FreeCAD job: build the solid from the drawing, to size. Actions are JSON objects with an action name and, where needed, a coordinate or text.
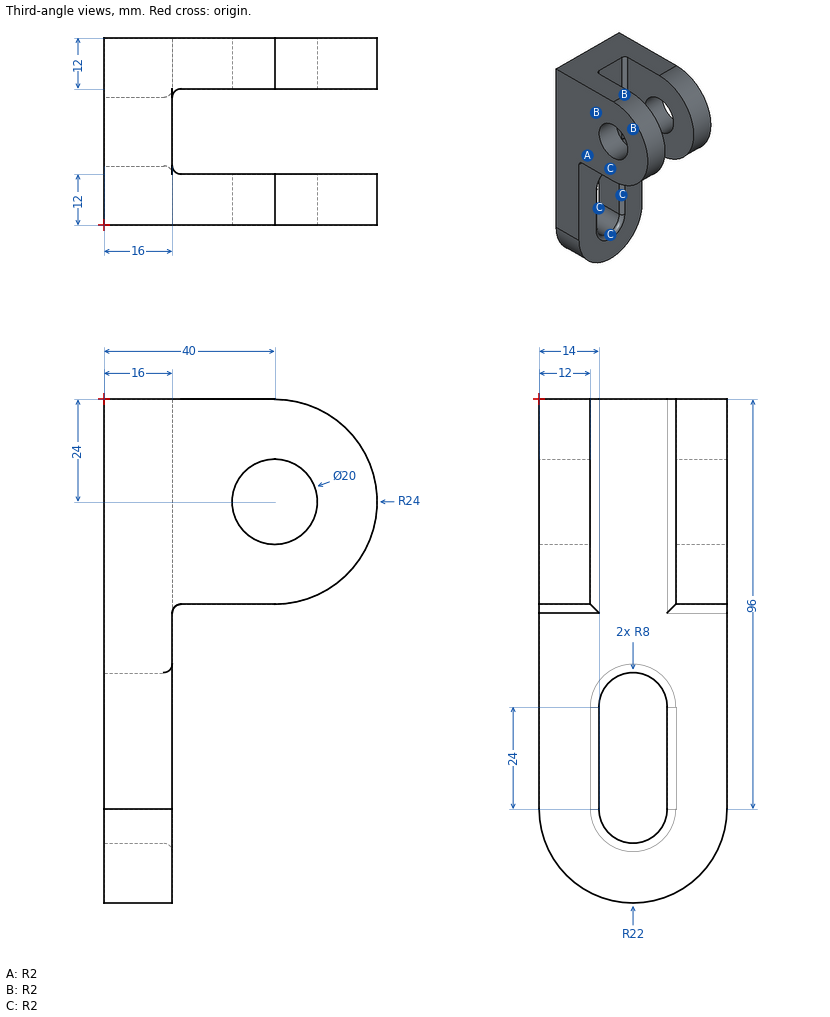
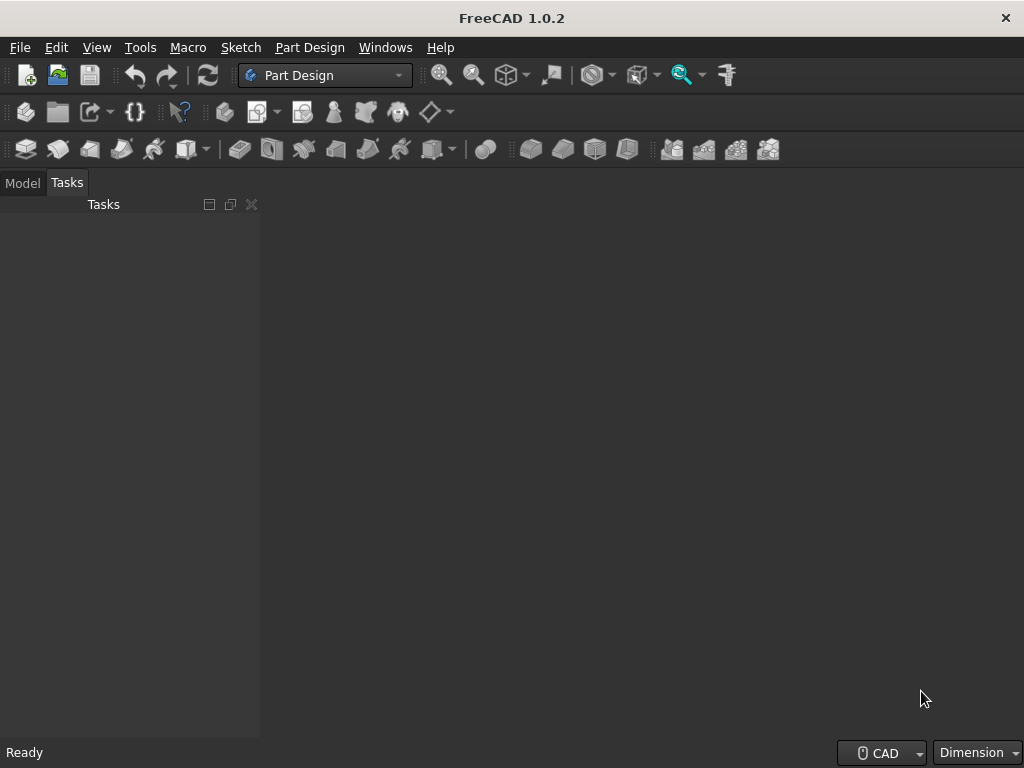
{"action": "left_click", "coordinate": [26, 76]}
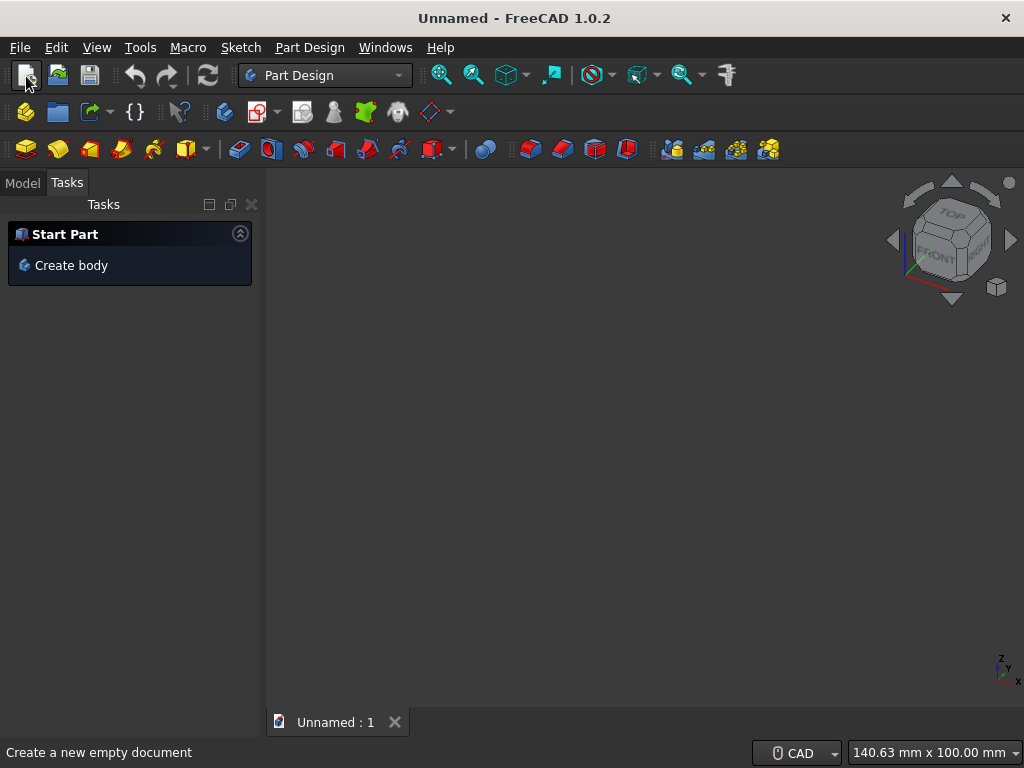
{"action": "left_click", "coordinate": [258, 112]}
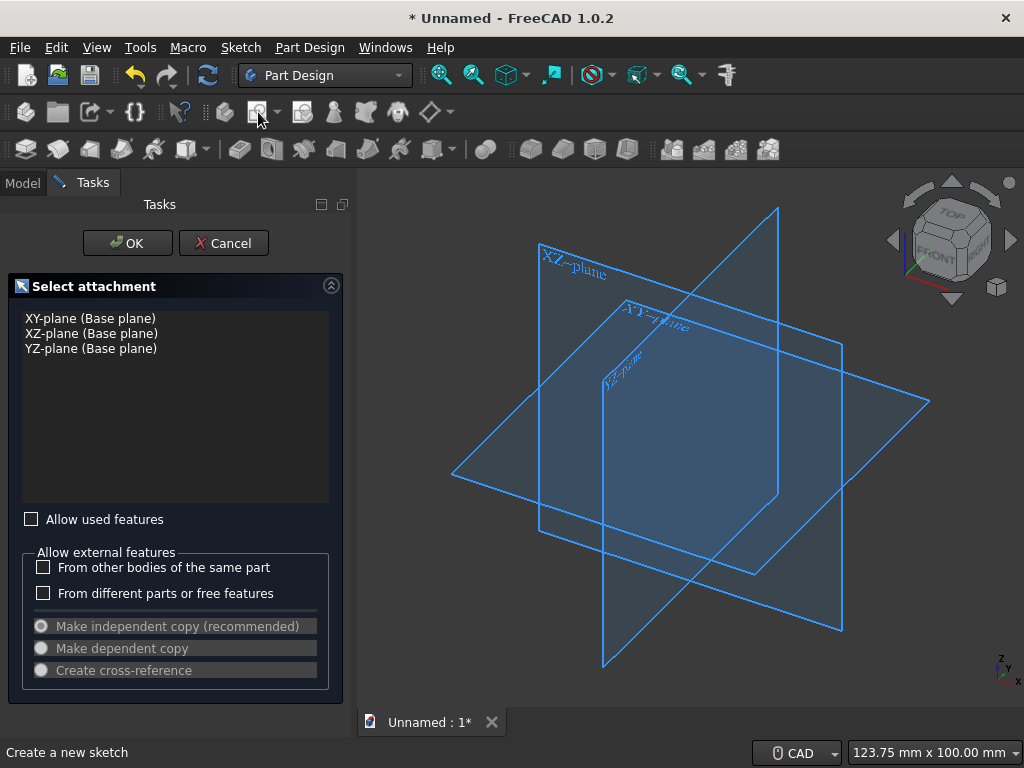
{"action": "left_click", "coordinate": [82, 348]}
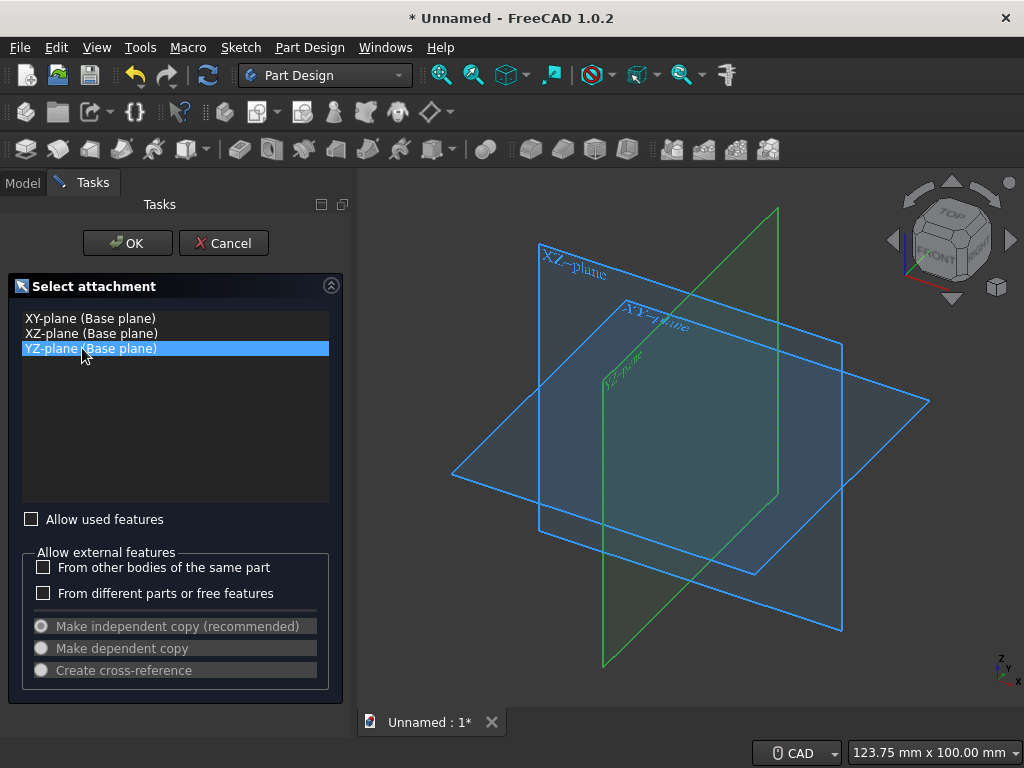
{"action": "left_click", "coordinate": [128, 243]}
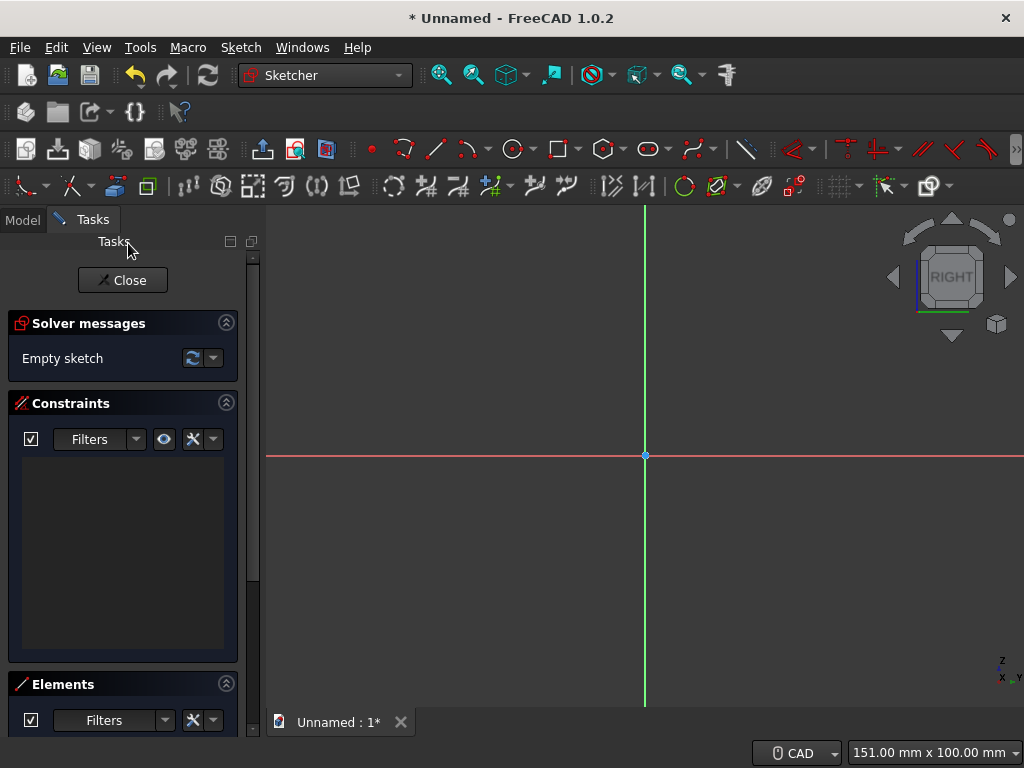
{"action": "scroll", "coordinate": [430, 233], "scroll_direction": "down", "scroll_amount": 4}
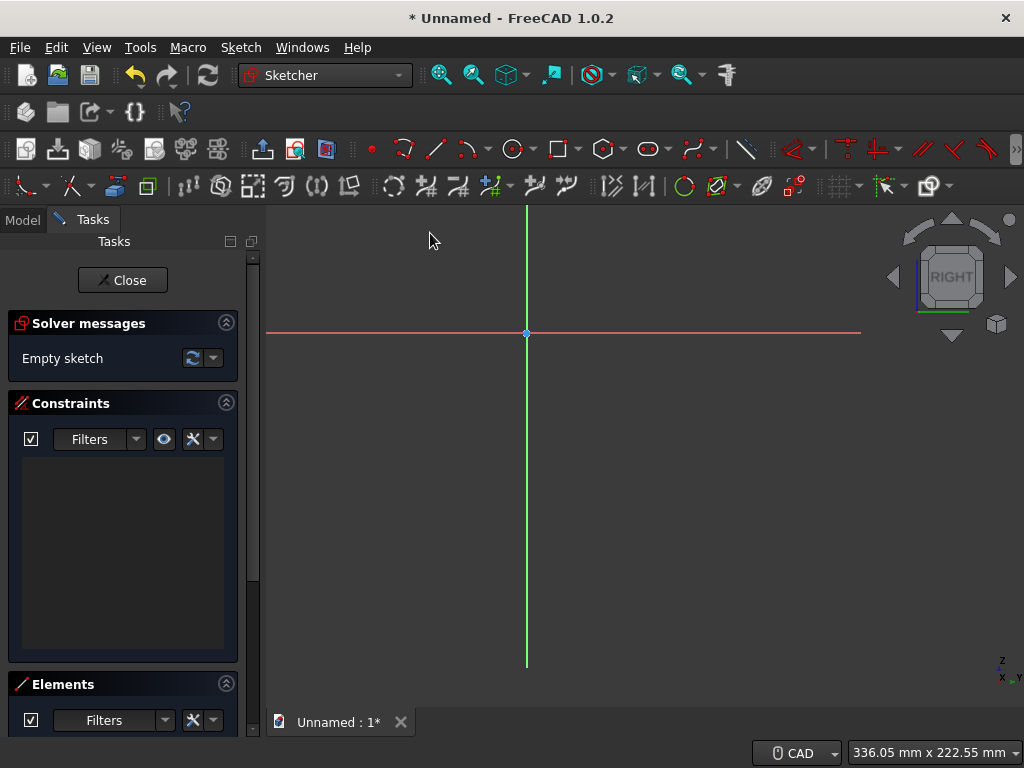
{"action": "left_click", "coordinate": [404, 150]}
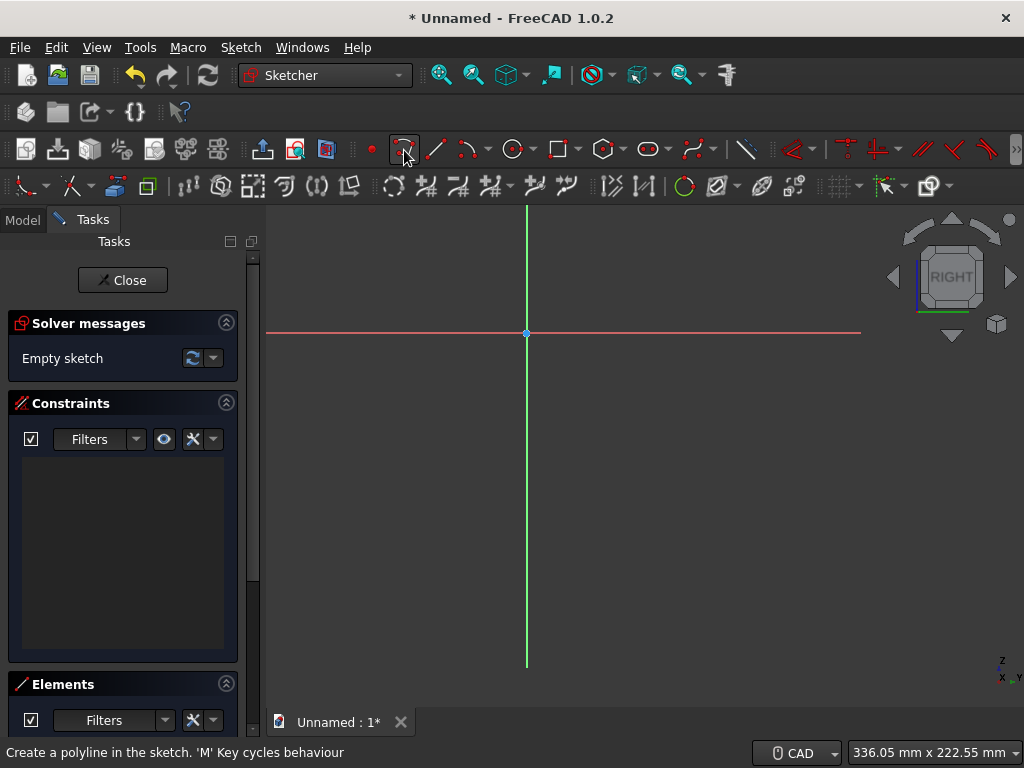
{"action": "left_click", "coordinate": [626, 550]}
{"action": "left_click", "coordinate": [626, 333]}
{"action": "left_click", "coordinate": [527, 333]}
{"action": "left_click", "coordinate": [536, 550]}
{"action": "right_click", "coordinate": [536, 550]}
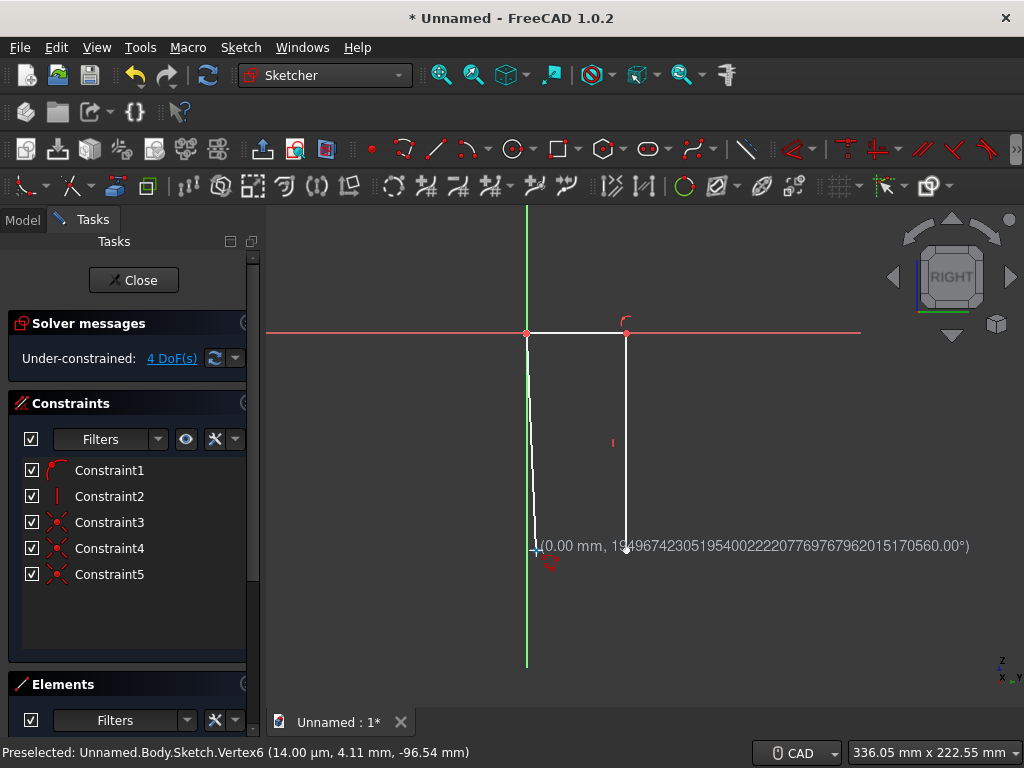
{"action": "left_click", "coordinate": [490, 150]}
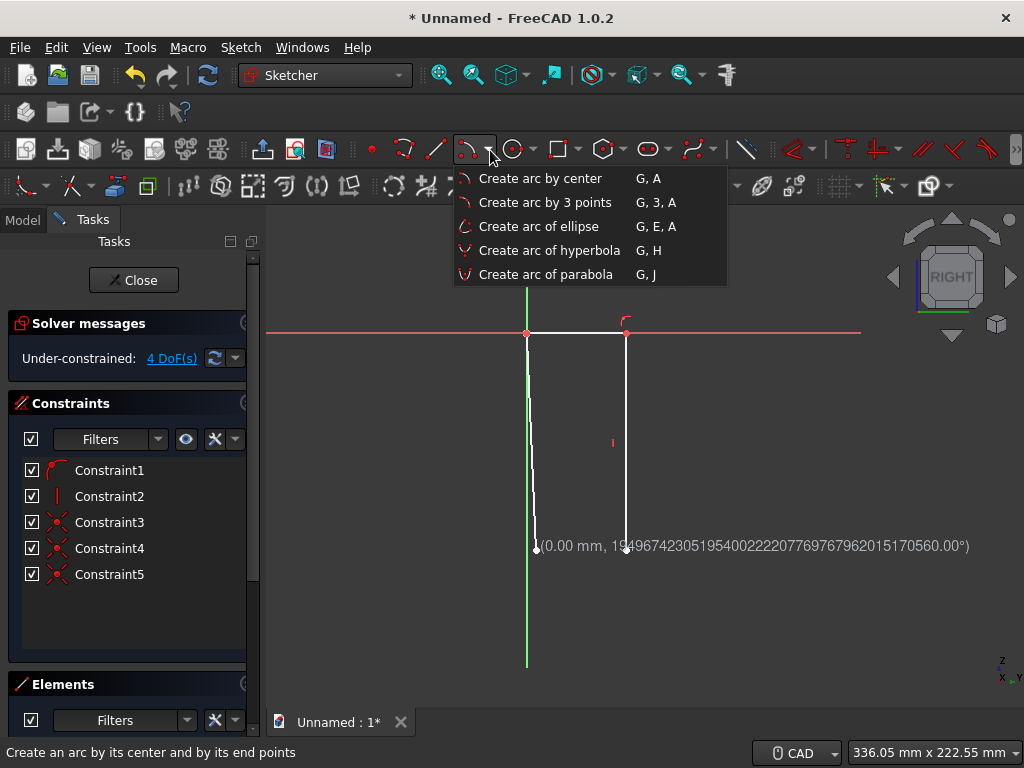
{"action": "left_click", "coordinate": [590, 202]}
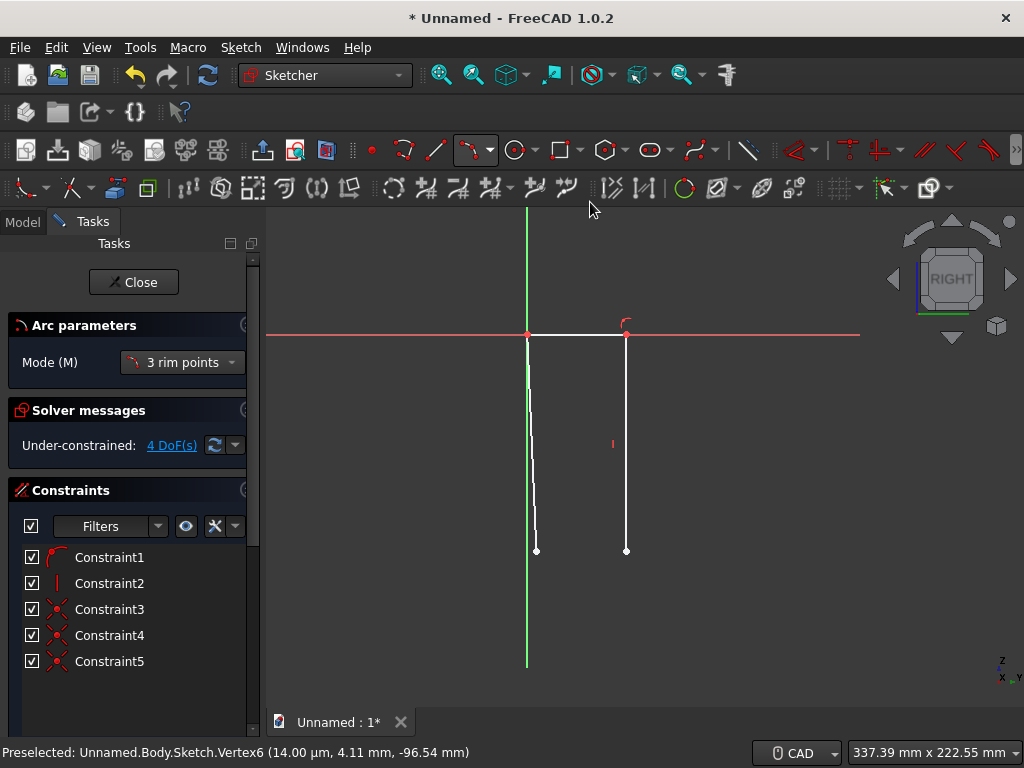
{"action": "left_click", "coordinate": [536, 552]}
{"action": "left_click", "coordinate": [626, 552]}
{"action": "left_click", "coordinate": [577, 600]}
{"action": "key", "text": "Escape"}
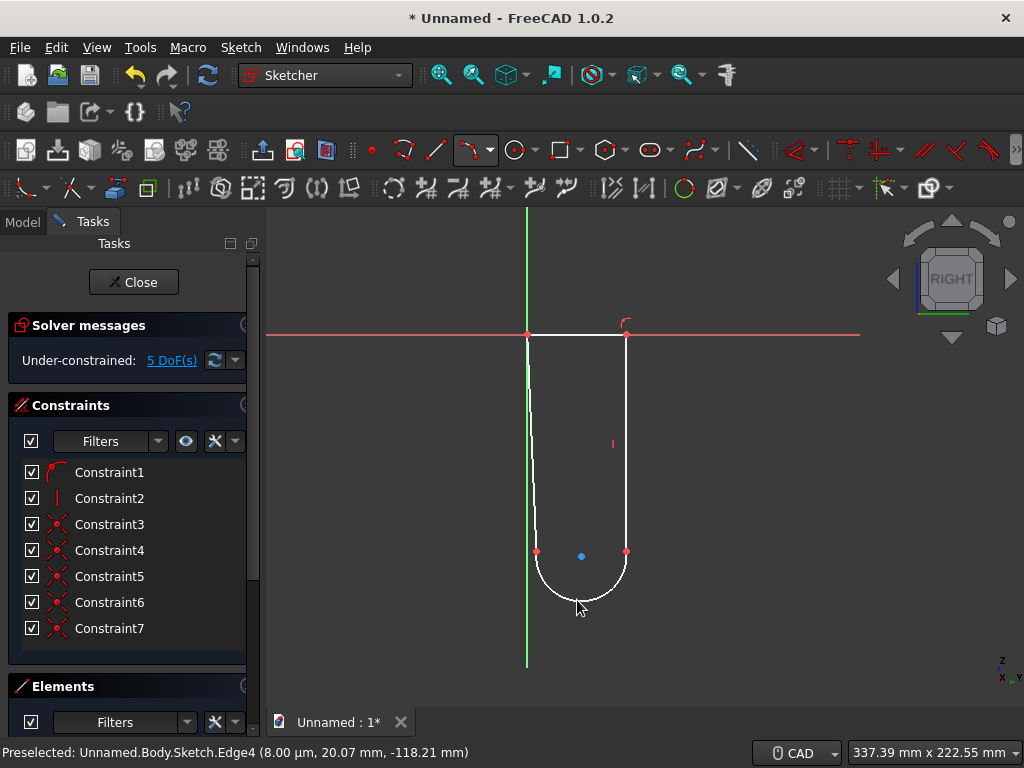
{"action": "left_click", "coordinate": [626, 487]}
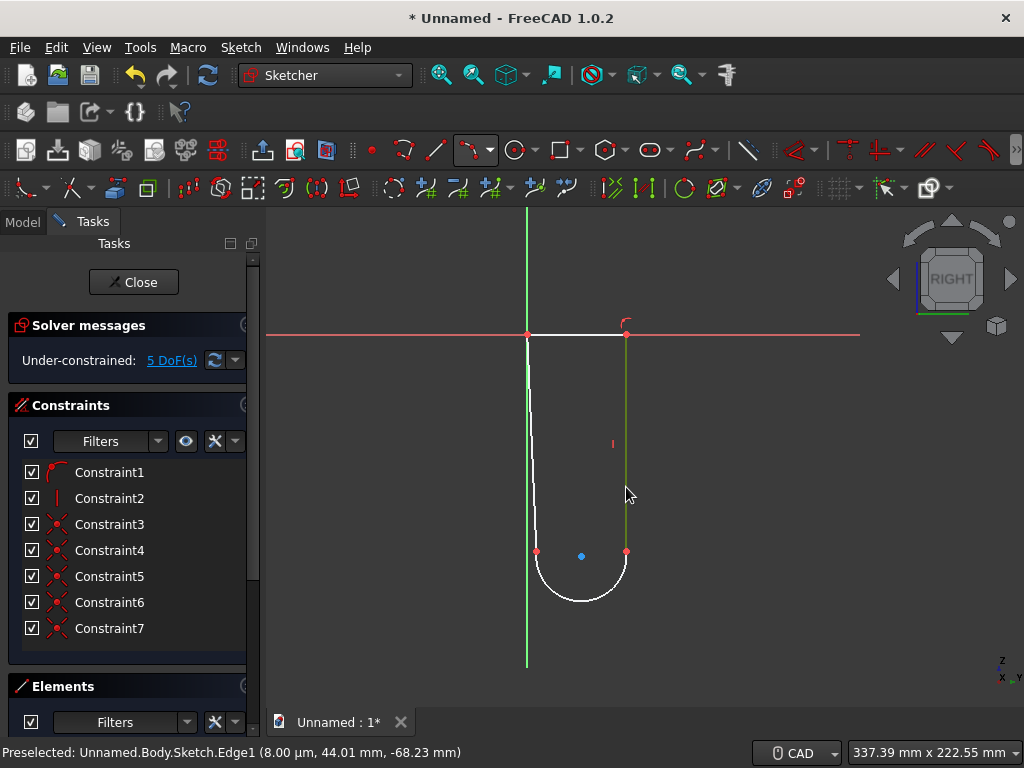
{"action": "left_click", "coordinate": [553, 592]}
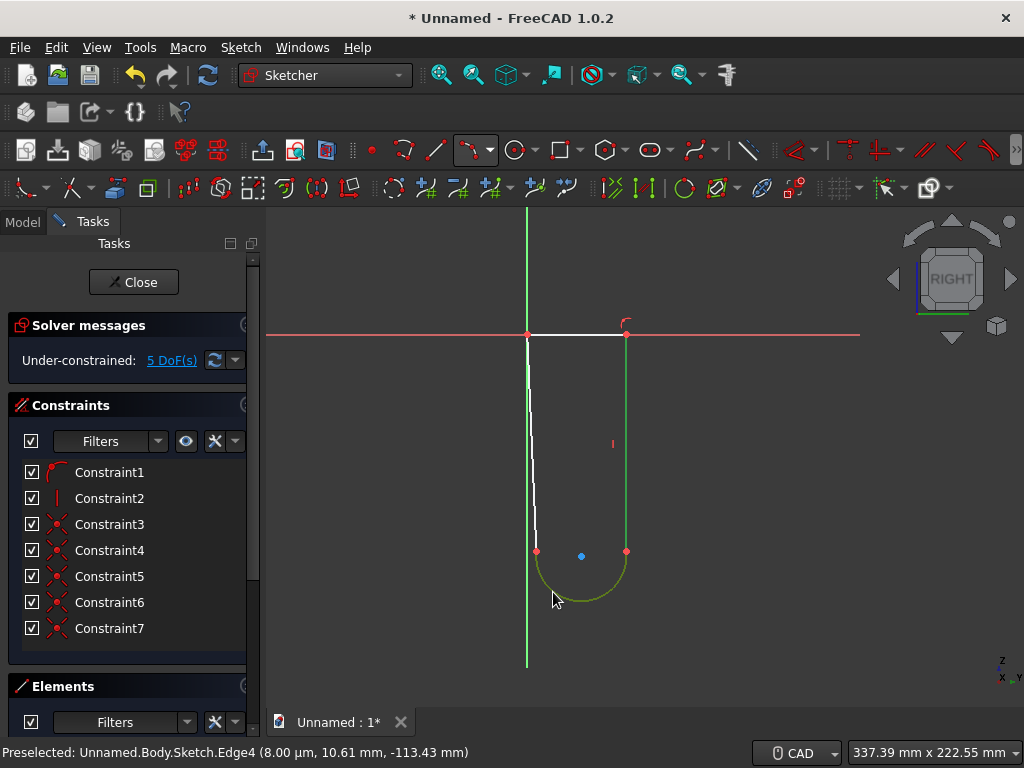
{"action": "left_click", "coordinate": [990, 150]}